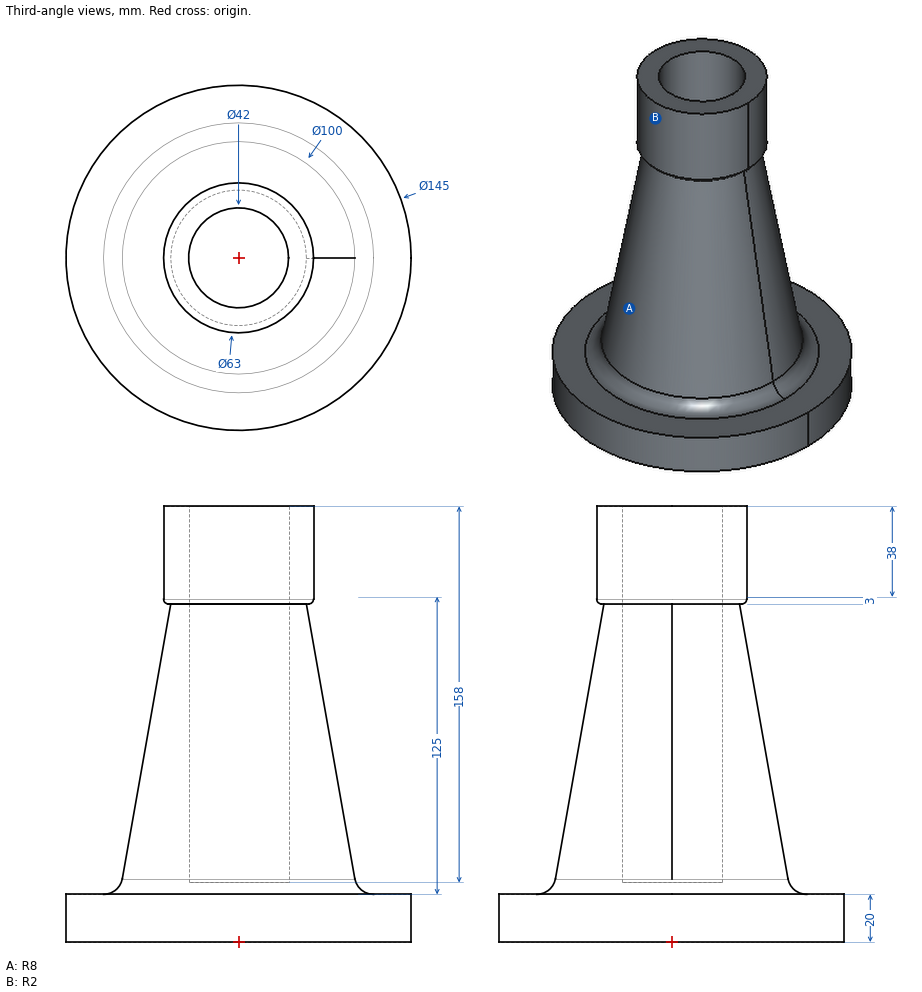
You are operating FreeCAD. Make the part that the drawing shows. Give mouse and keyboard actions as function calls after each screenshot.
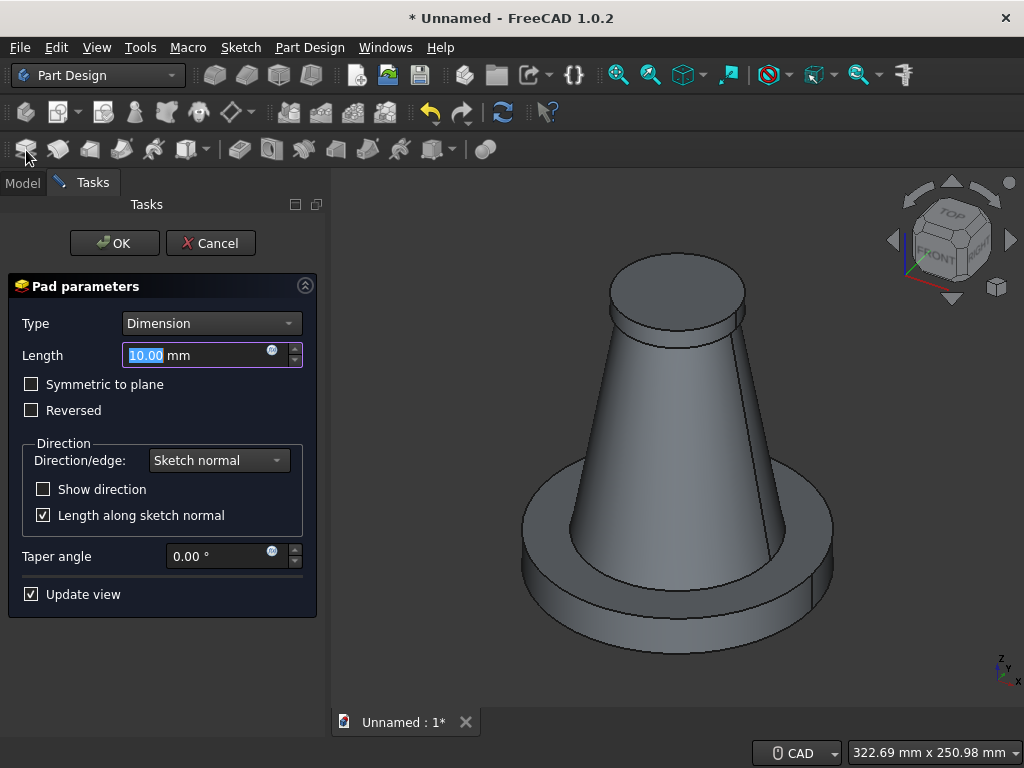
click(212, 324)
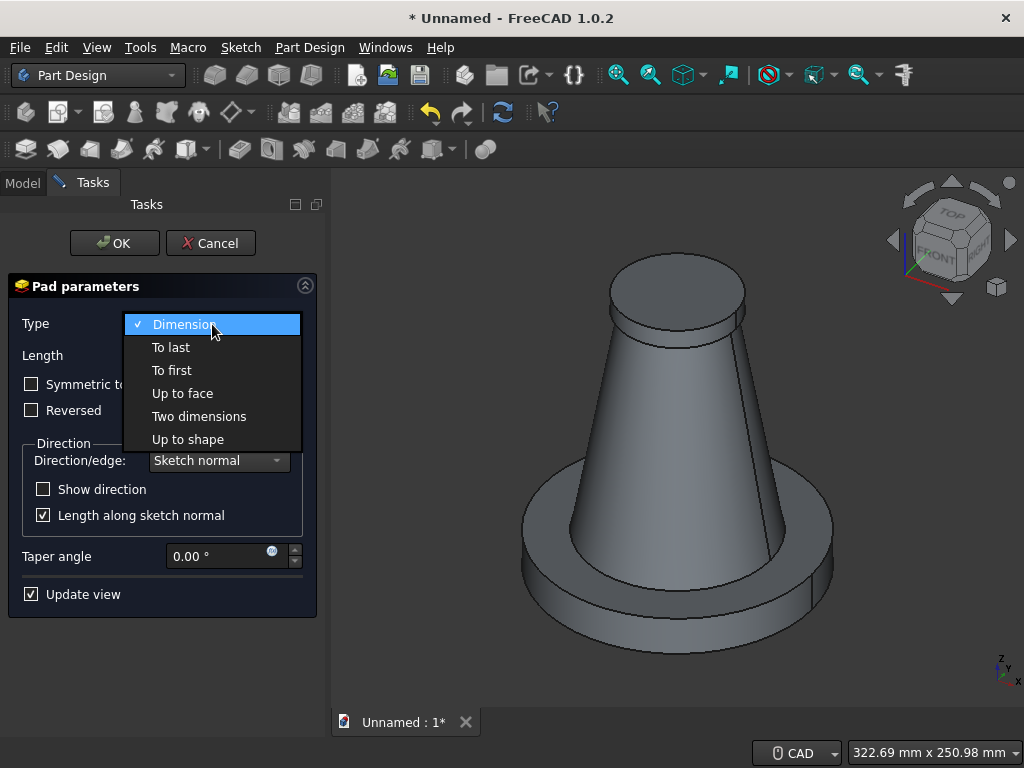
click(212, 416)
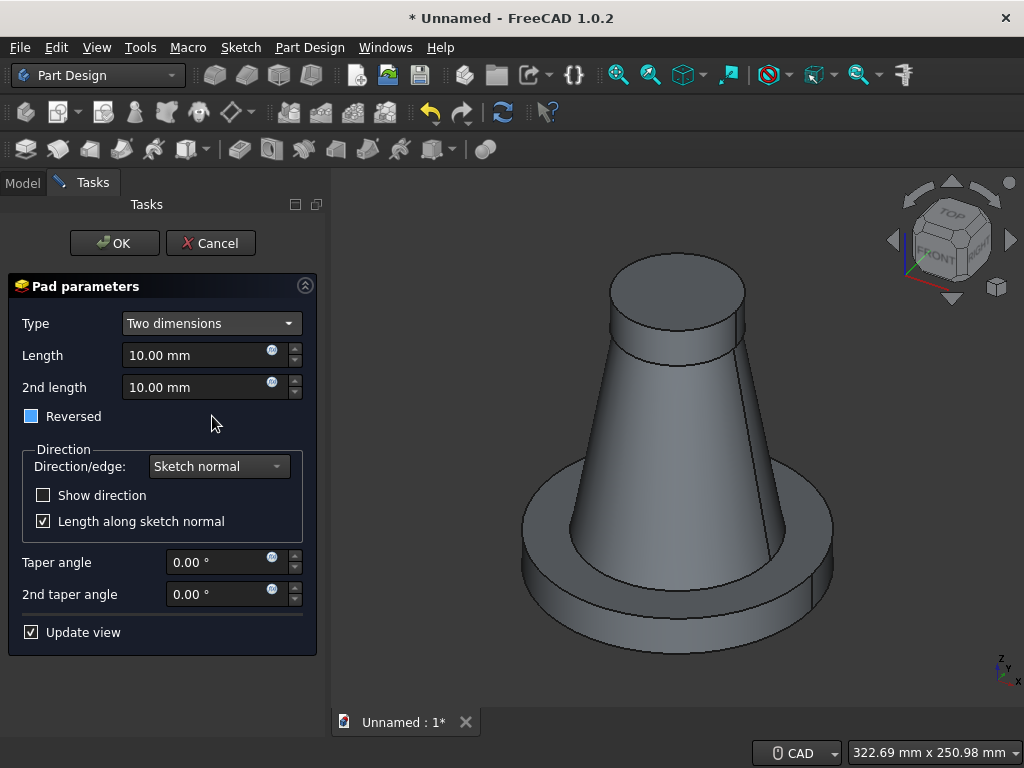
triple_click(204, 355)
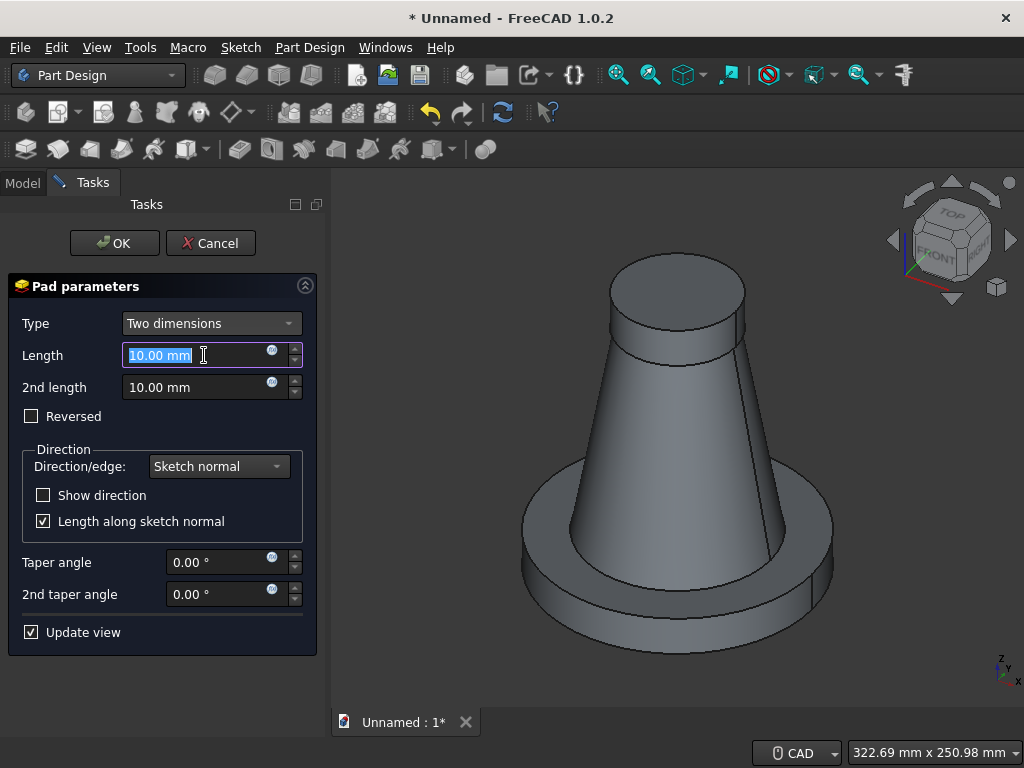
text(38)
key(Tab)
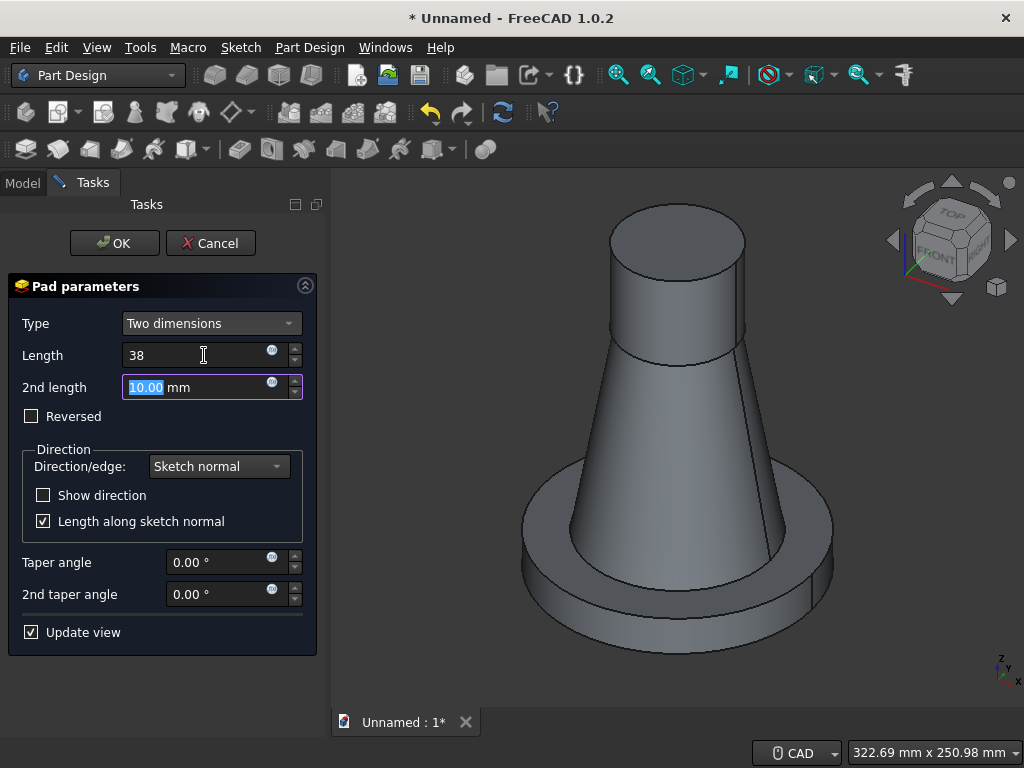
text(3)
key(Tab)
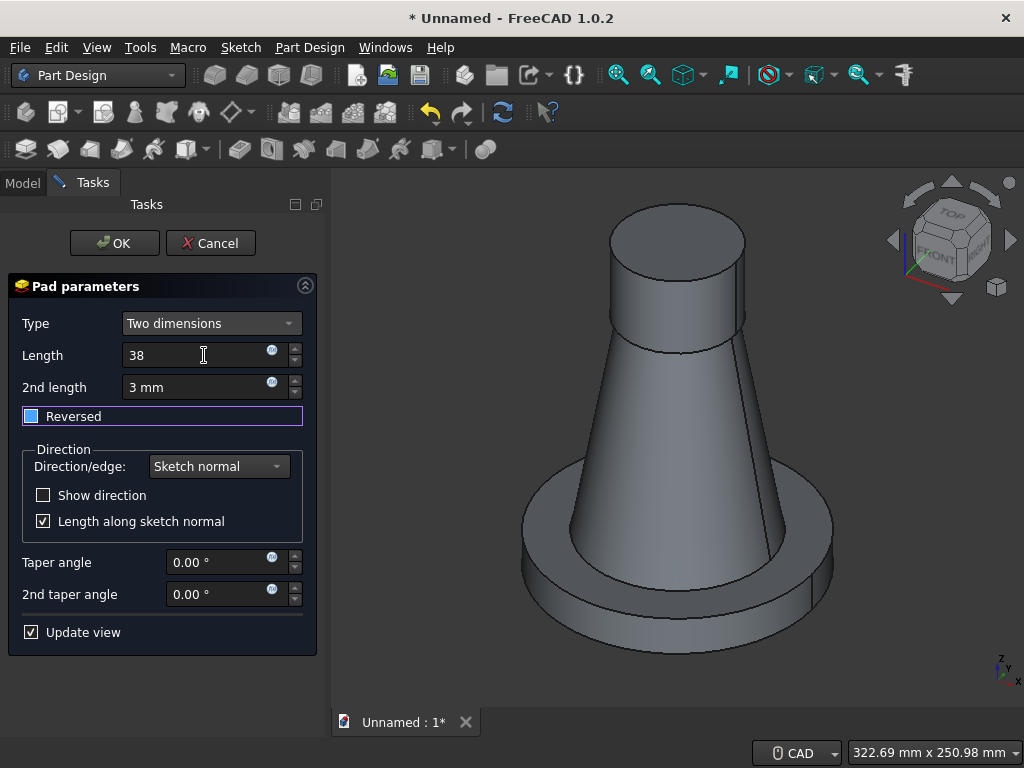
click(115, 243)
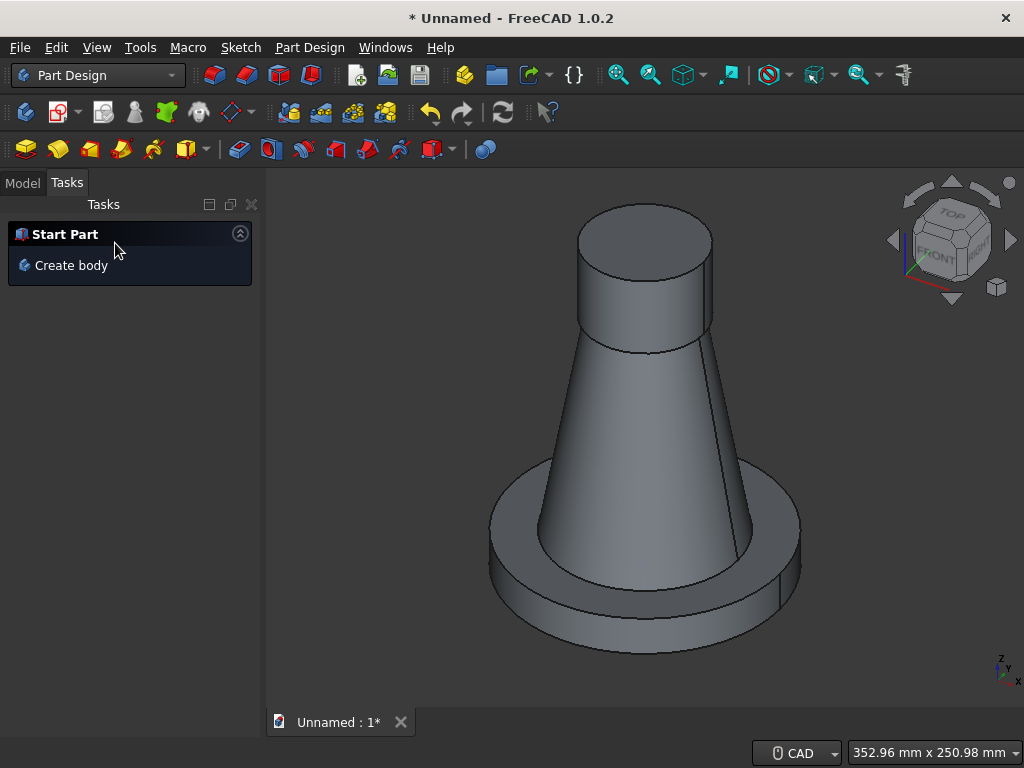
key(v)
key(f)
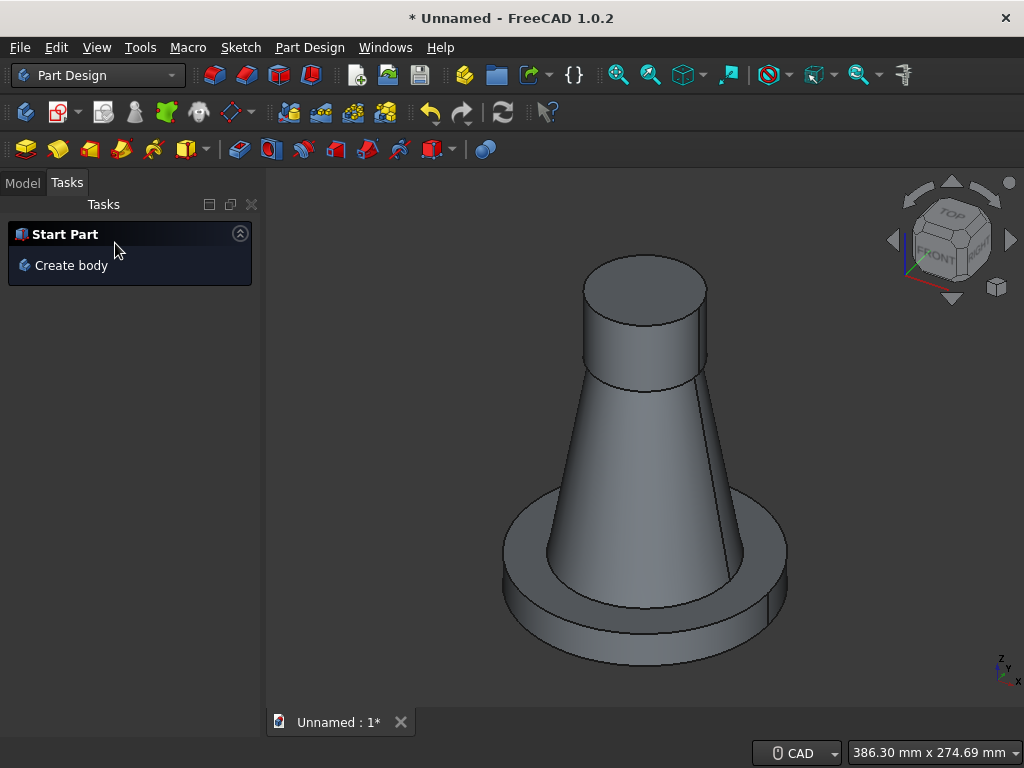
click(645, 289)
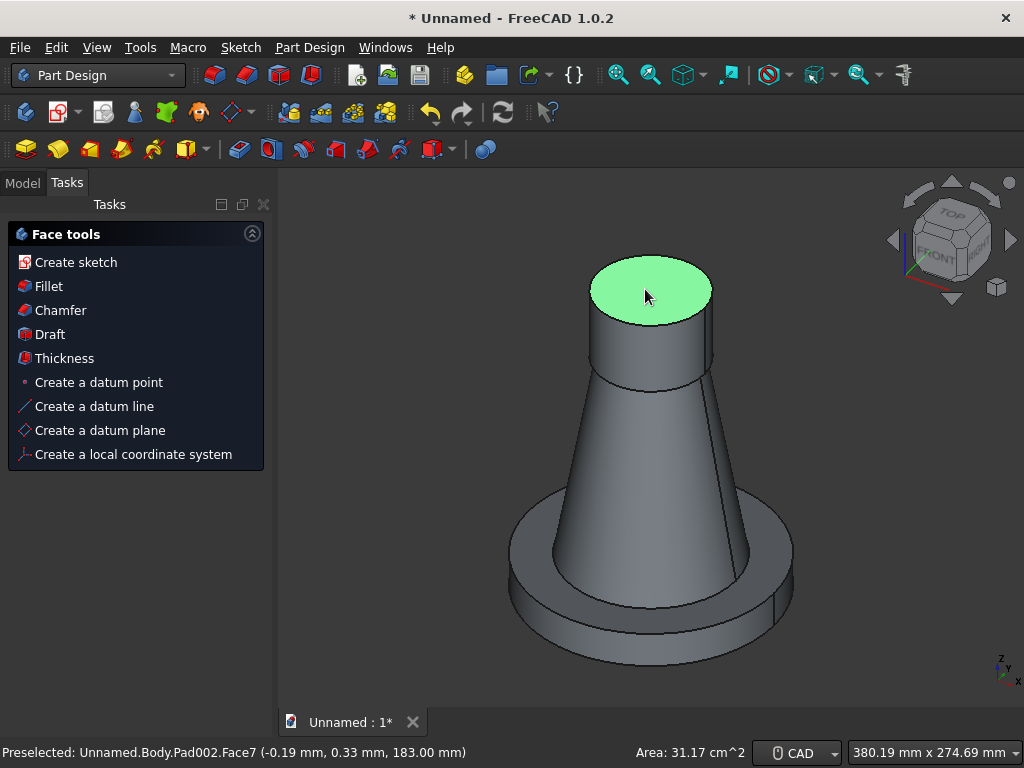
click(58, 112)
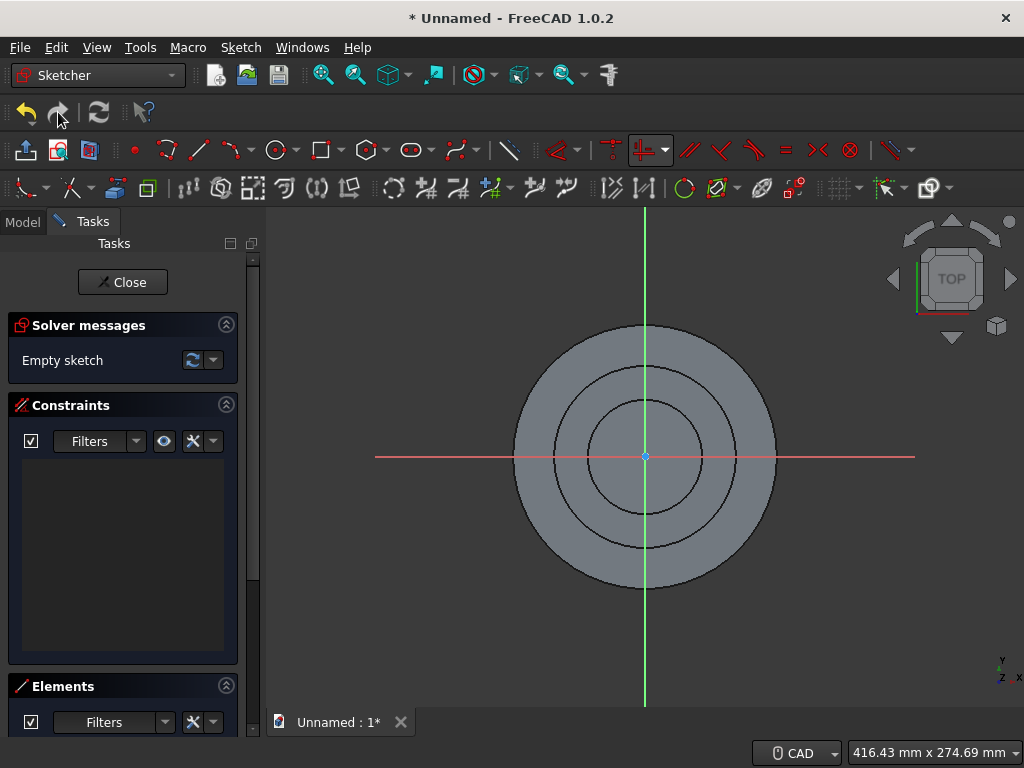
scroll(667, 457, up, 7)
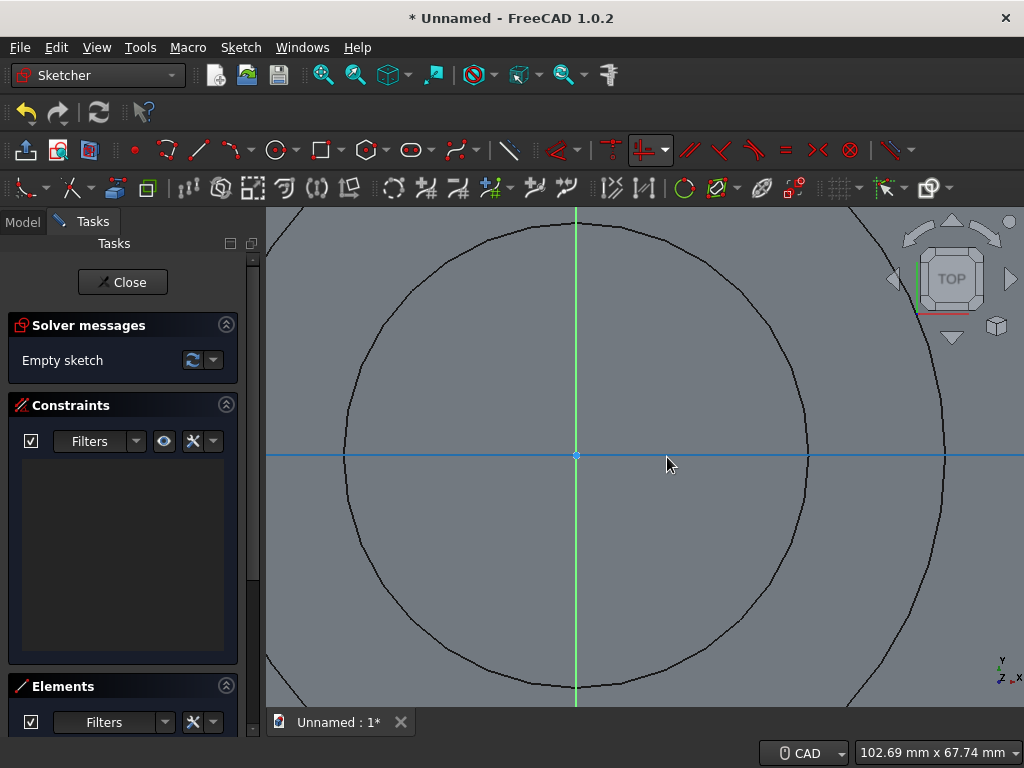
click(276, 150)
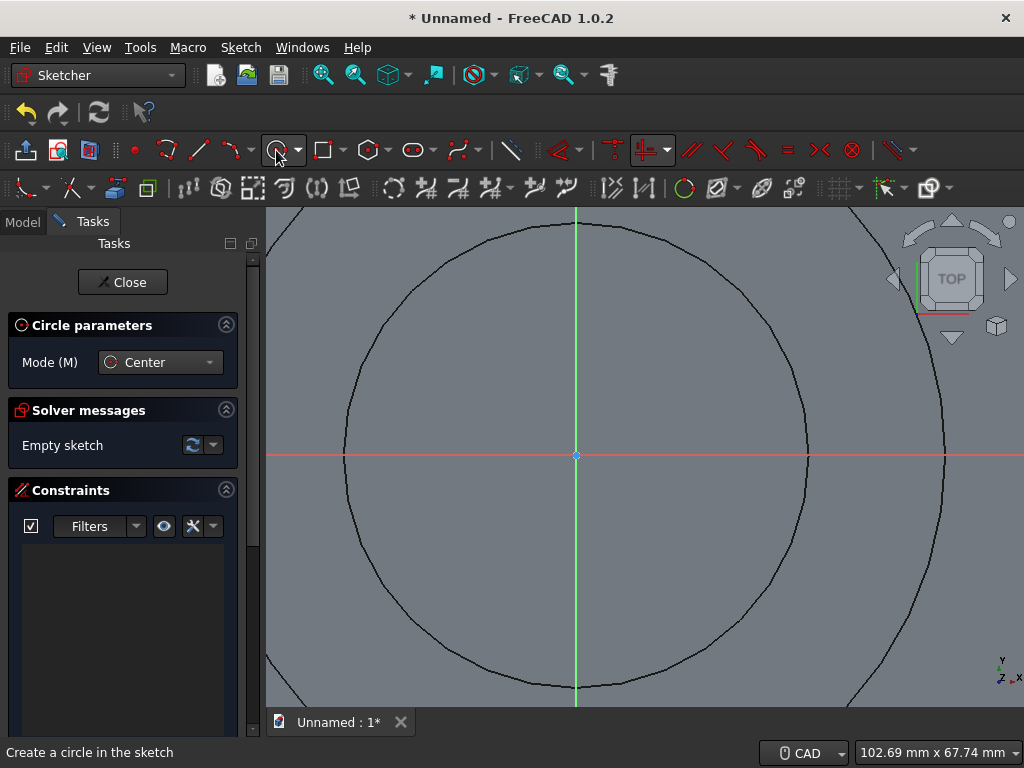
click(576, 455)
click(686, 346)
key(Escape)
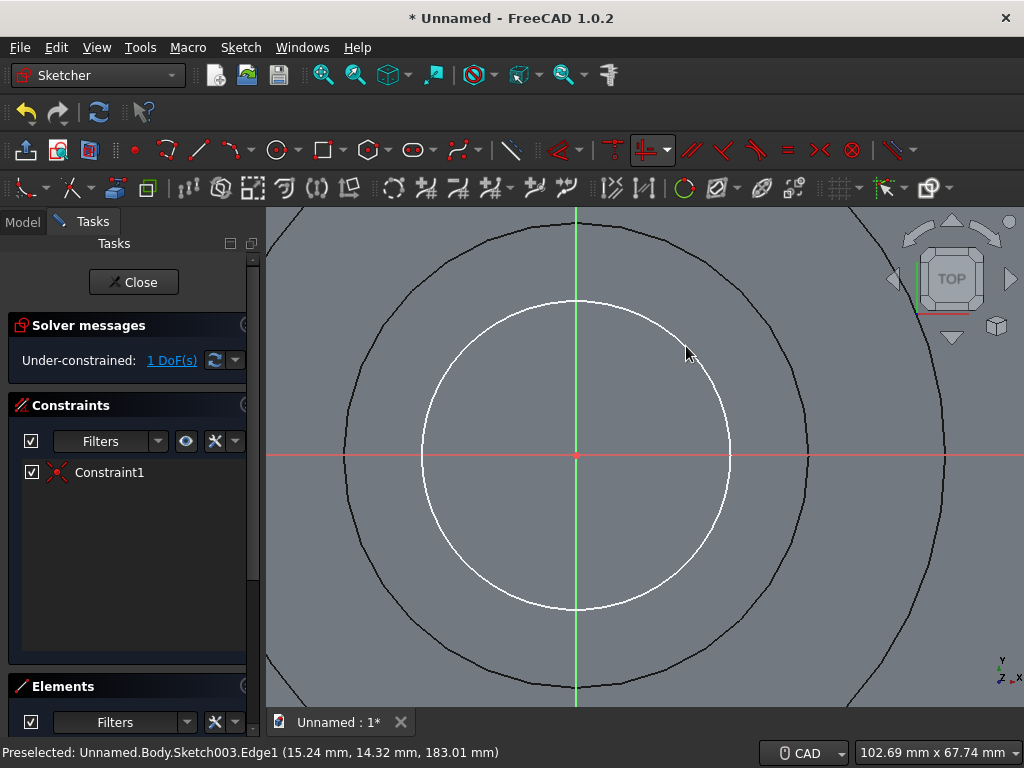
key(d)